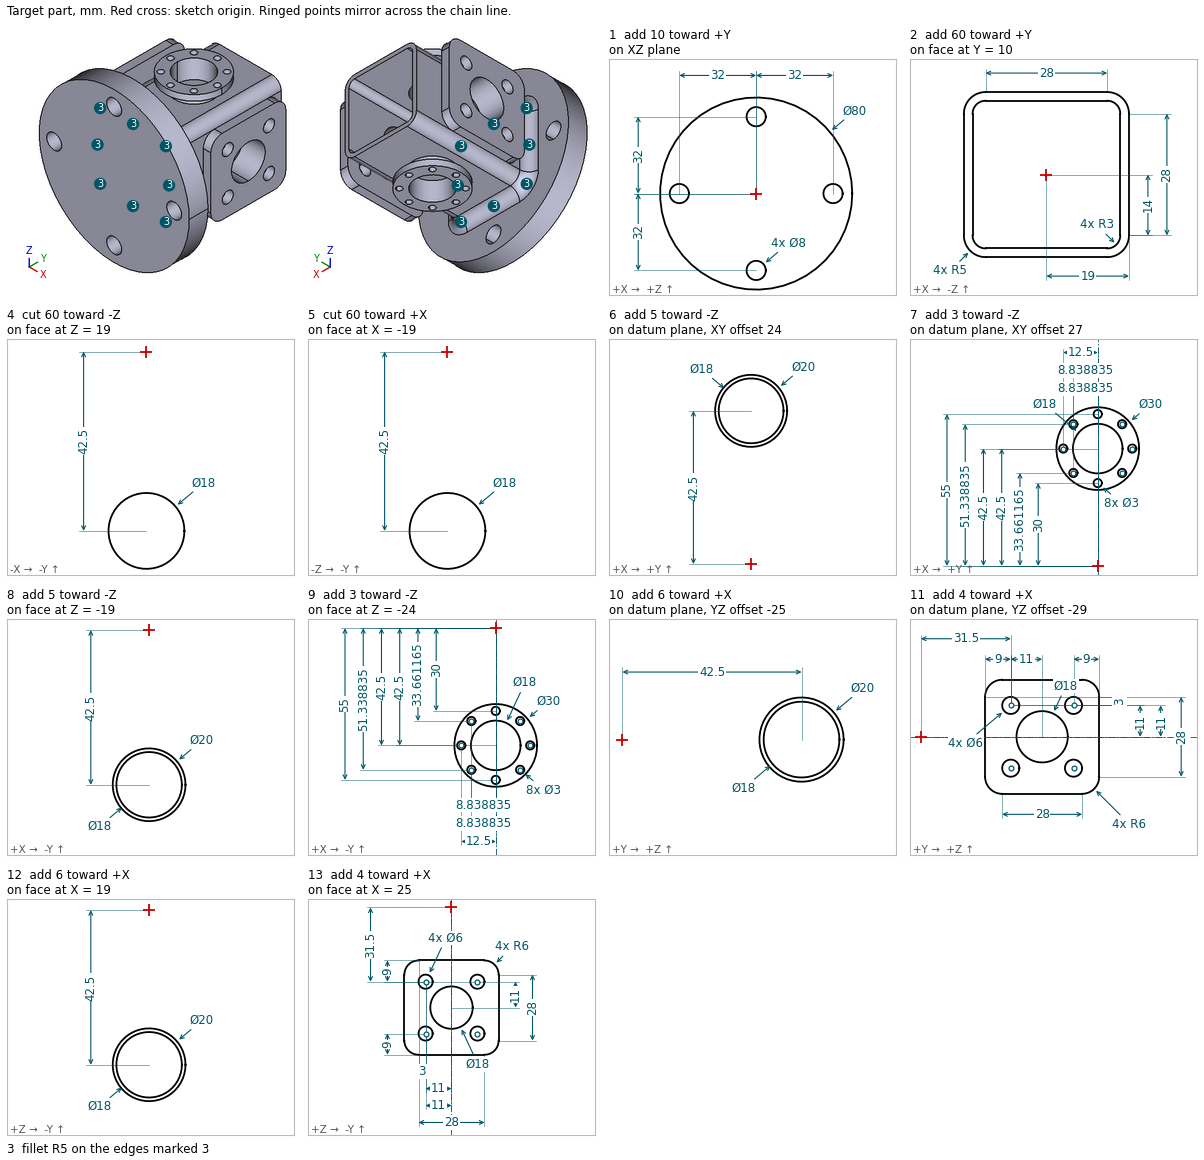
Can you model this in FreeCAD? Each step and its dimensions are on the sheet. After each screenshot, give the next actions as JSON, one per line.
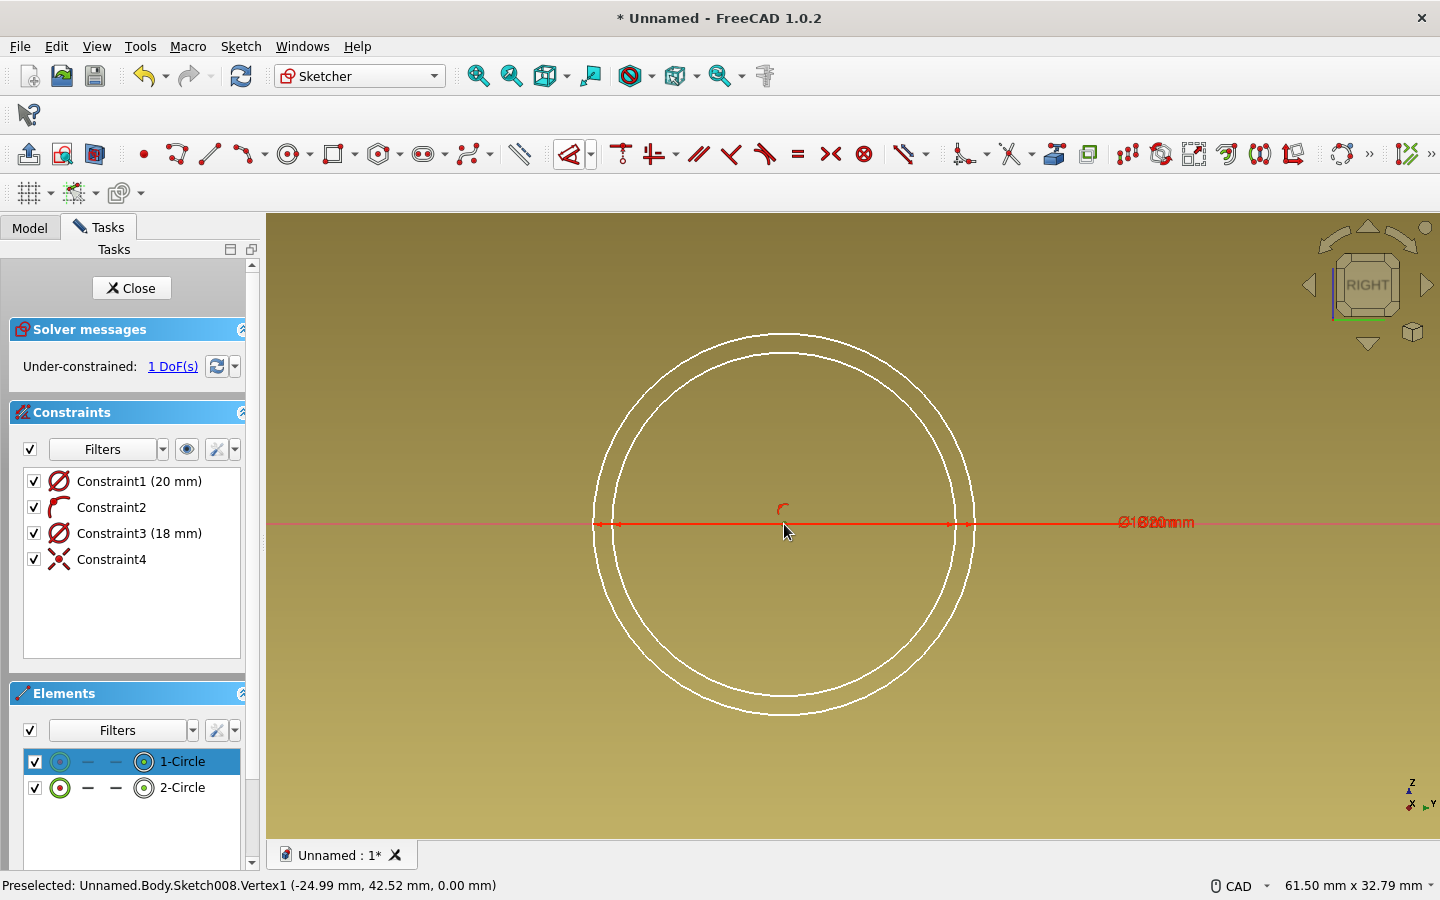
{"action": "key", "text": "l"}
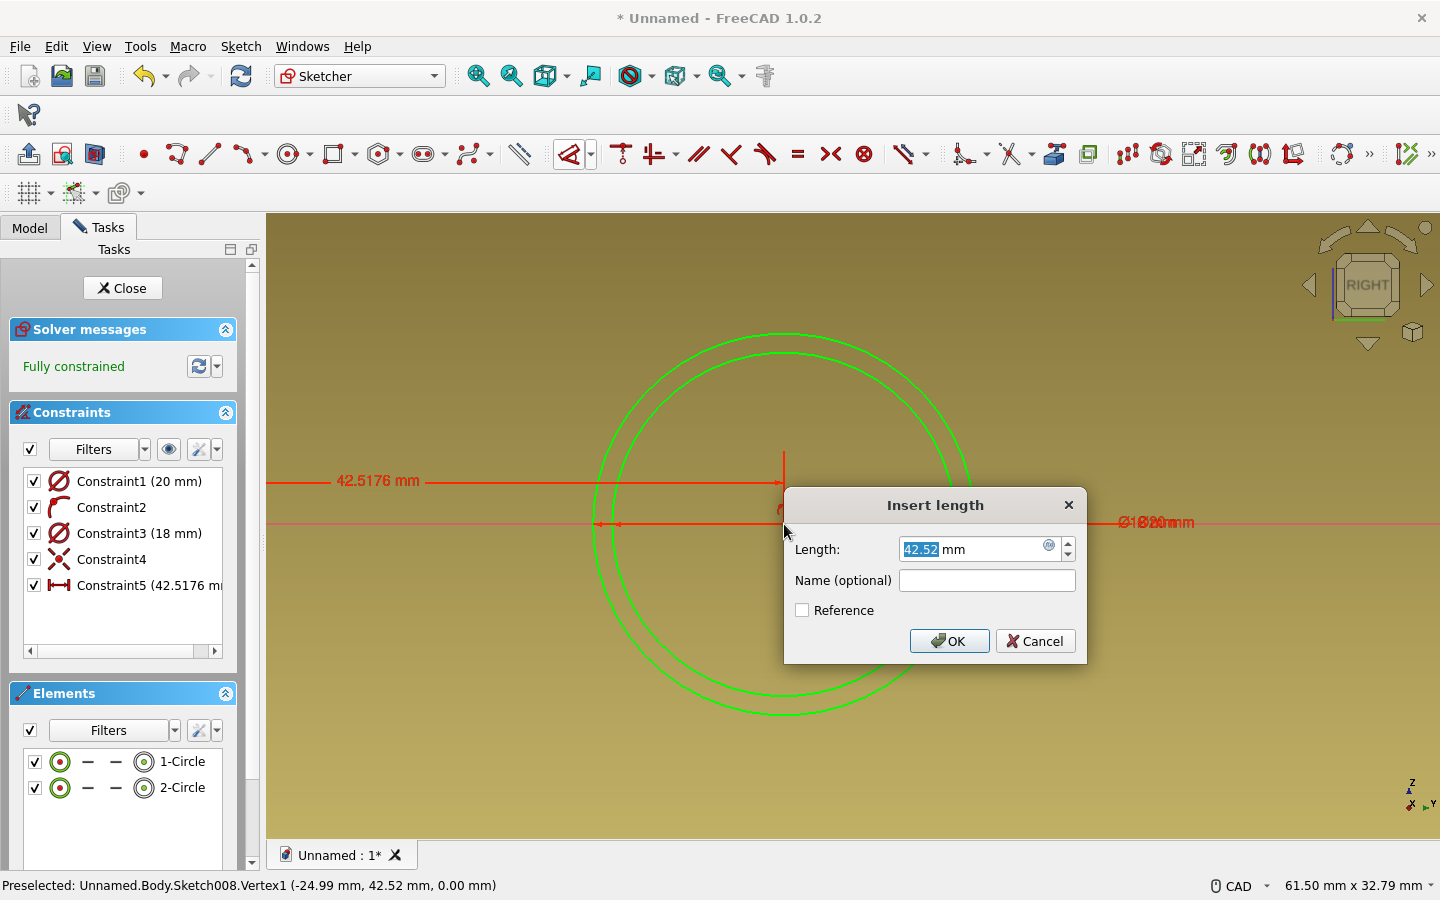
{"action": "type", "text": "42.5"}
{"action": "key", "text": "Return"}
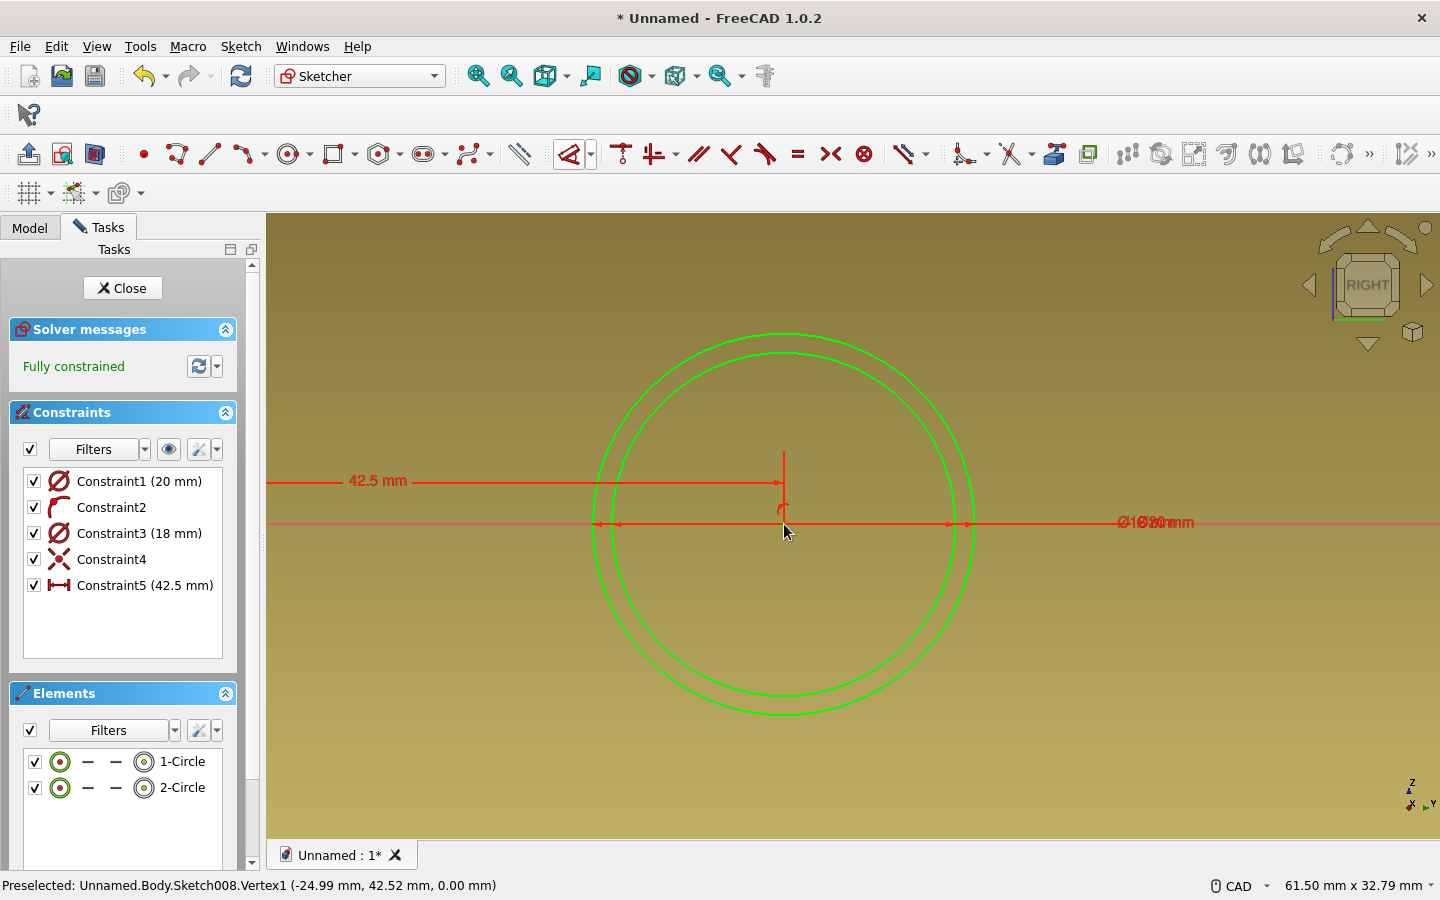
{"action": "left_click", "coordinate": [123, 288]}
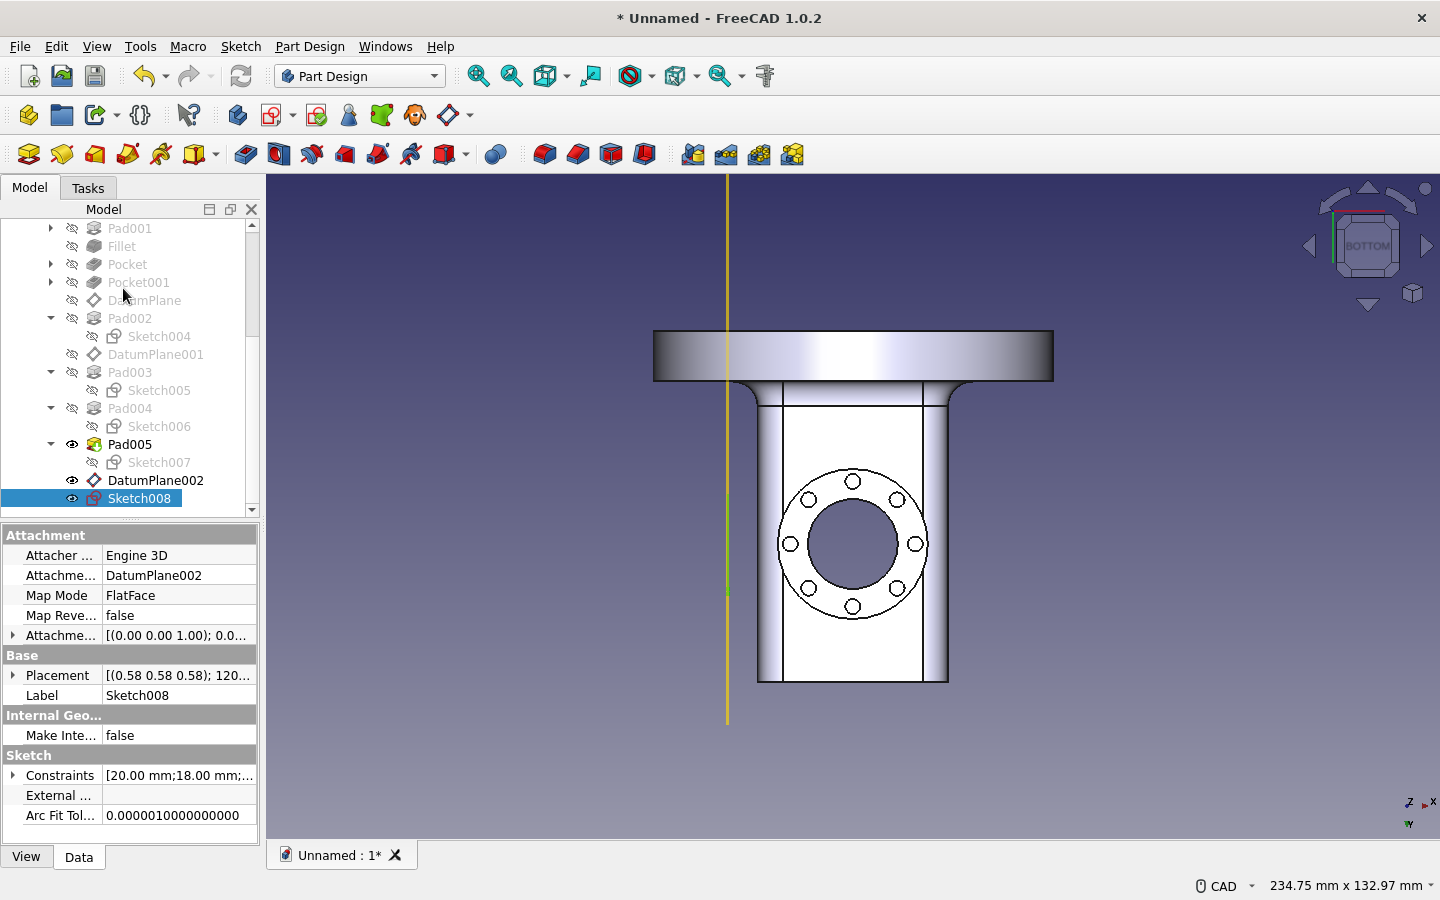
{"action": "left_click", "coordinate": [29, 154]}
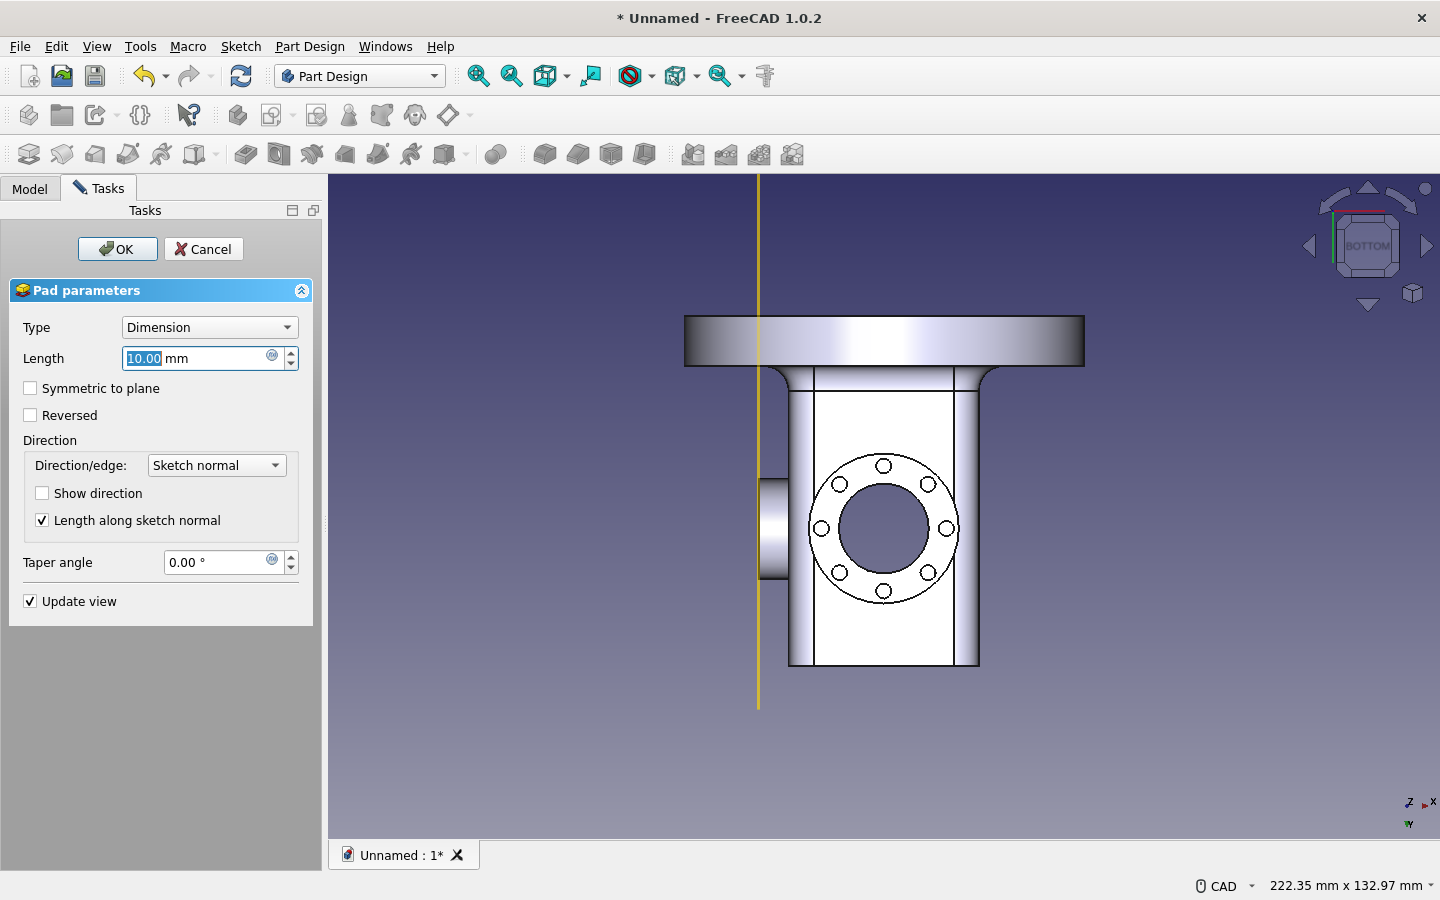
{"action": "type", "text": "6"}
{"action": "key", "text": "Tab"}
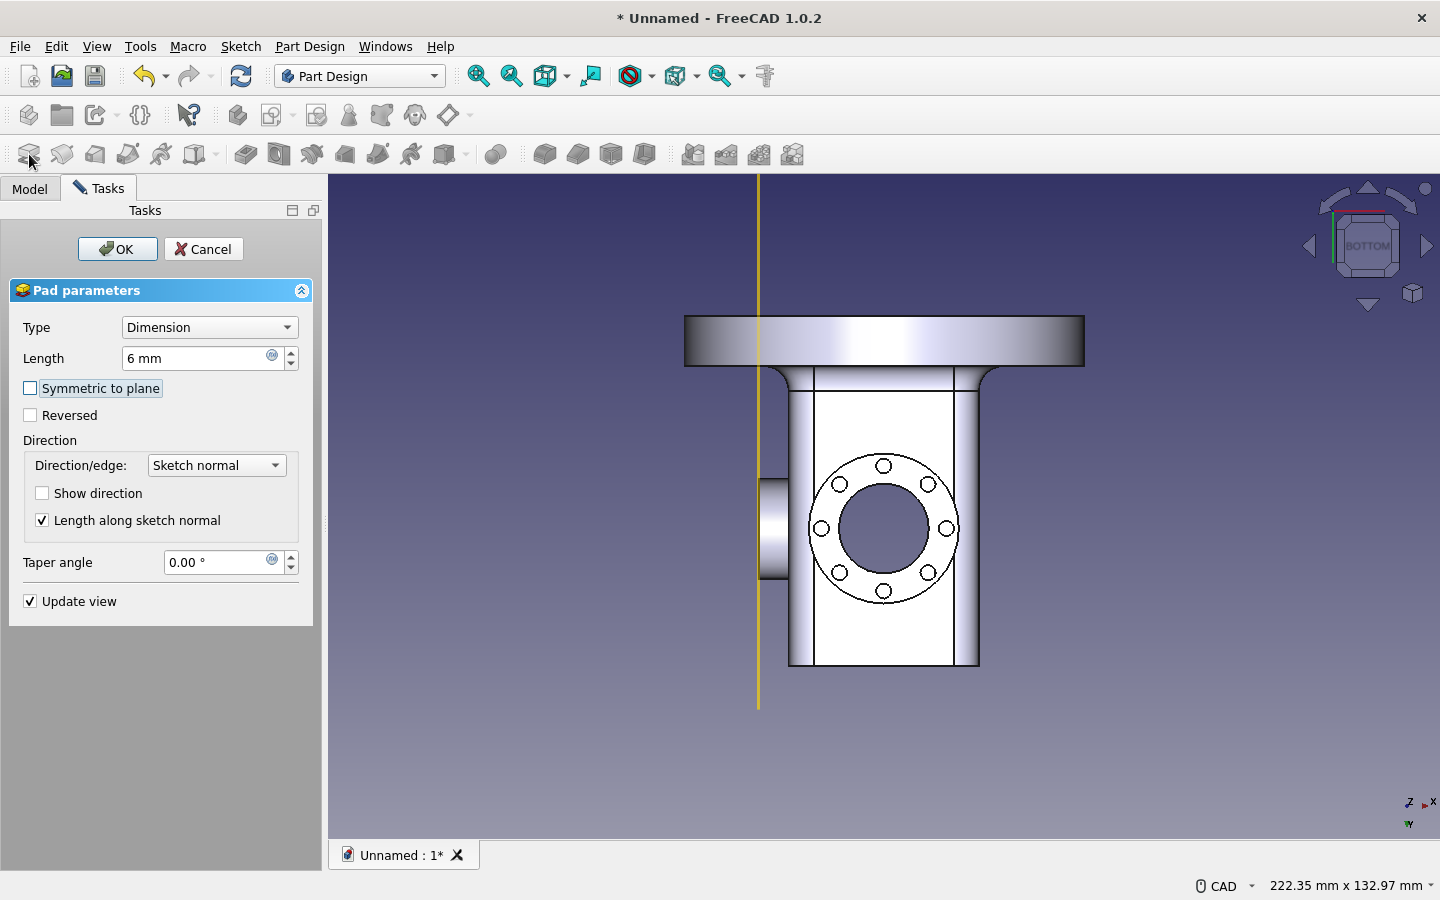
{"action": "left_click", "coordinate": [118, 249]}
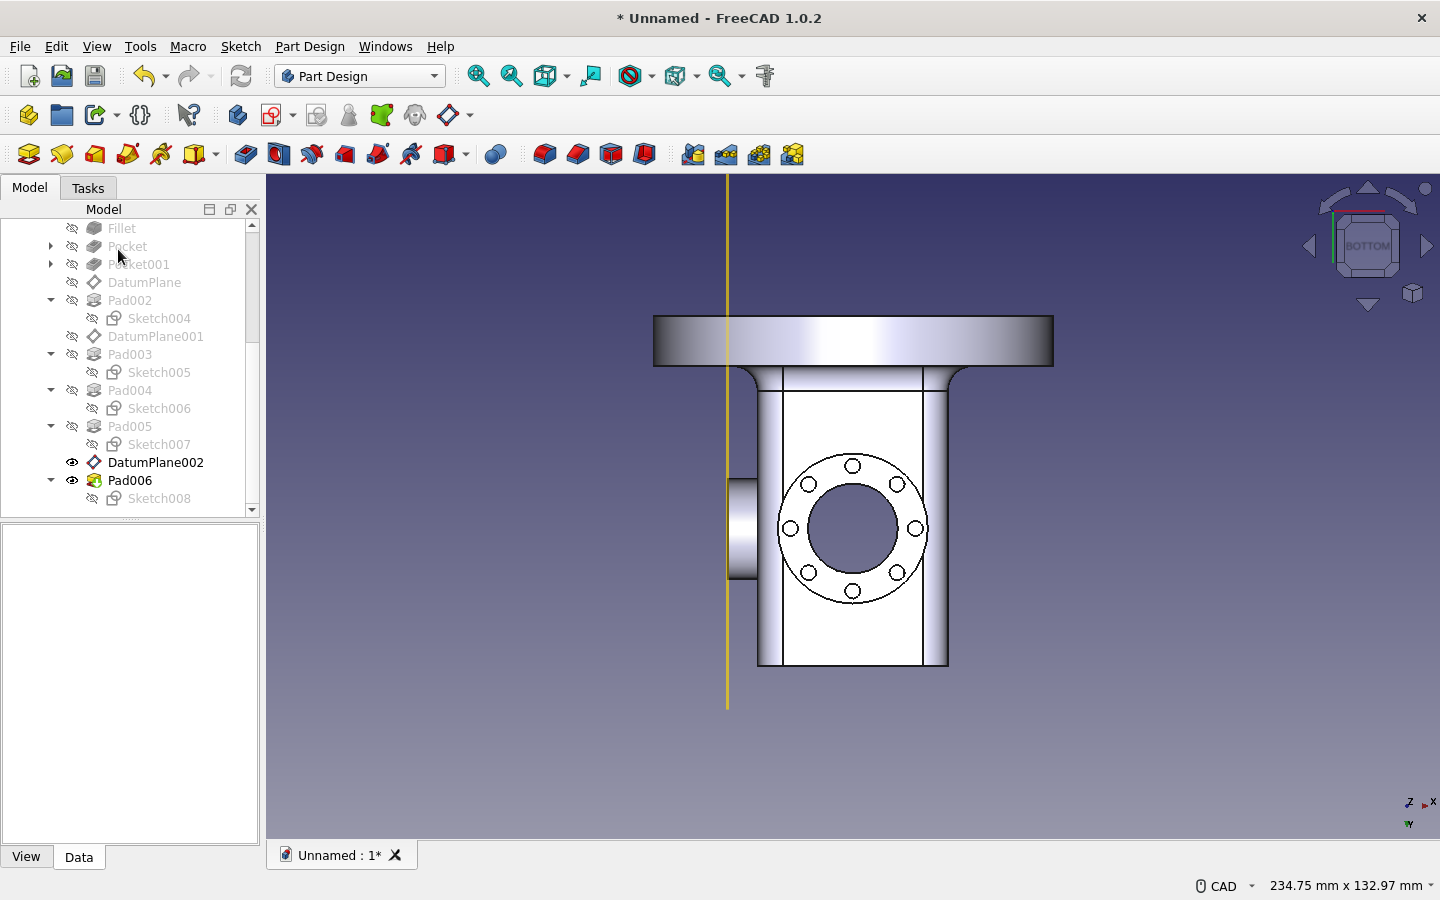
{"action": "left_click", "coordinate": [117, 462]}
{"action": "key", "text": "space"}